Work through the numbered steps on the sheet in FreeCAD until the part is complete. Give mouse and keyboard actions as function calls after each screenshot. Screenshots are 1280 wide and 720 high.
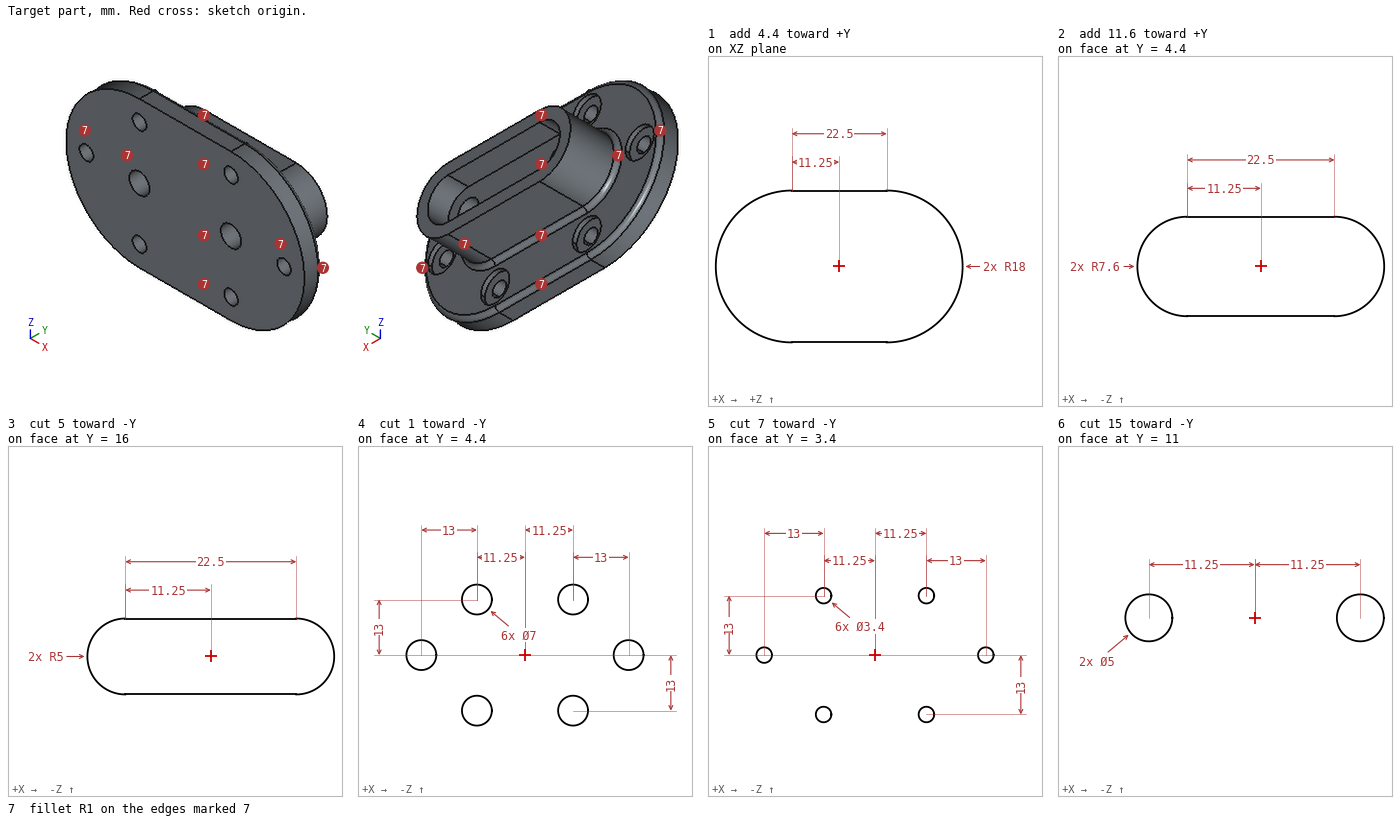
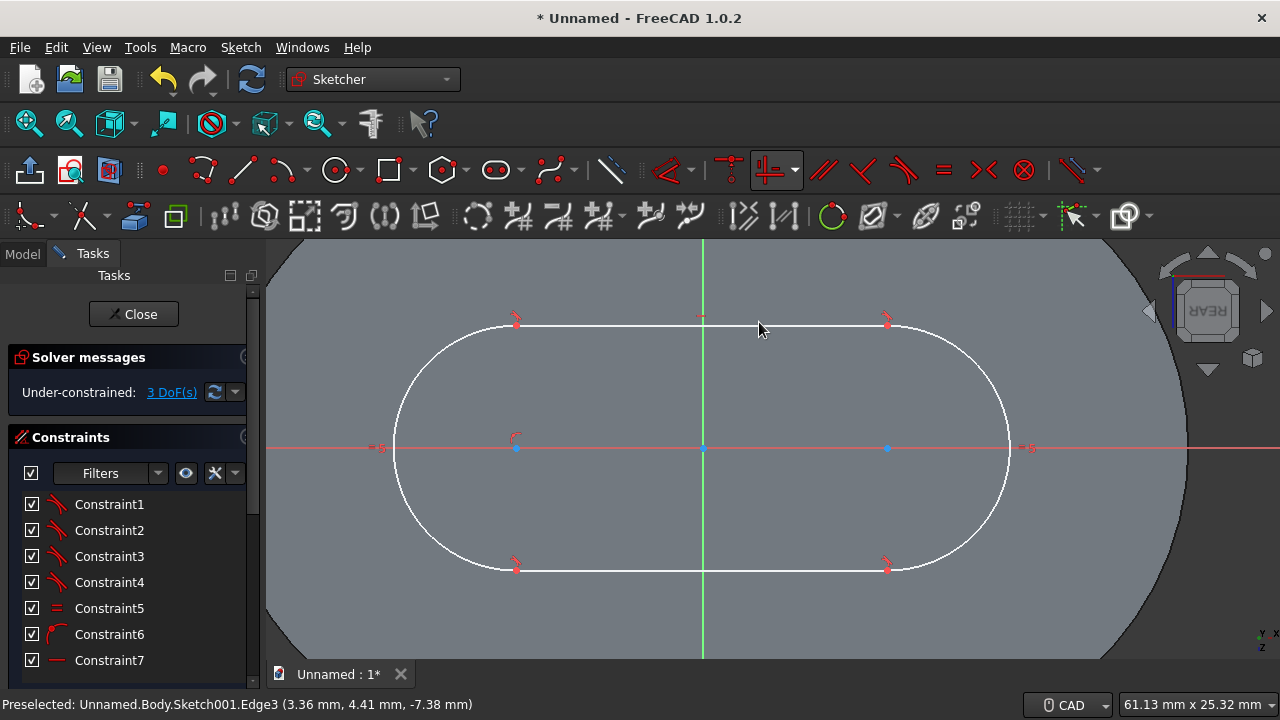
click(666, 170)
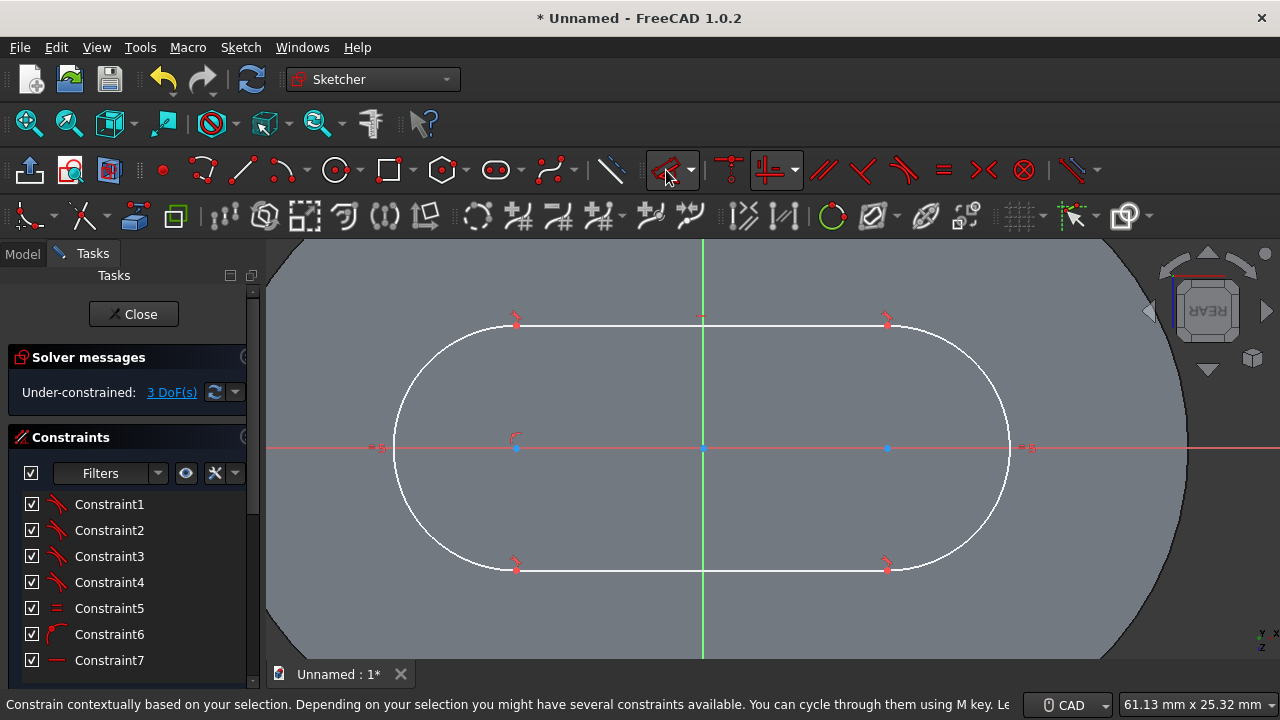
click(417, 376)
click(391, 357)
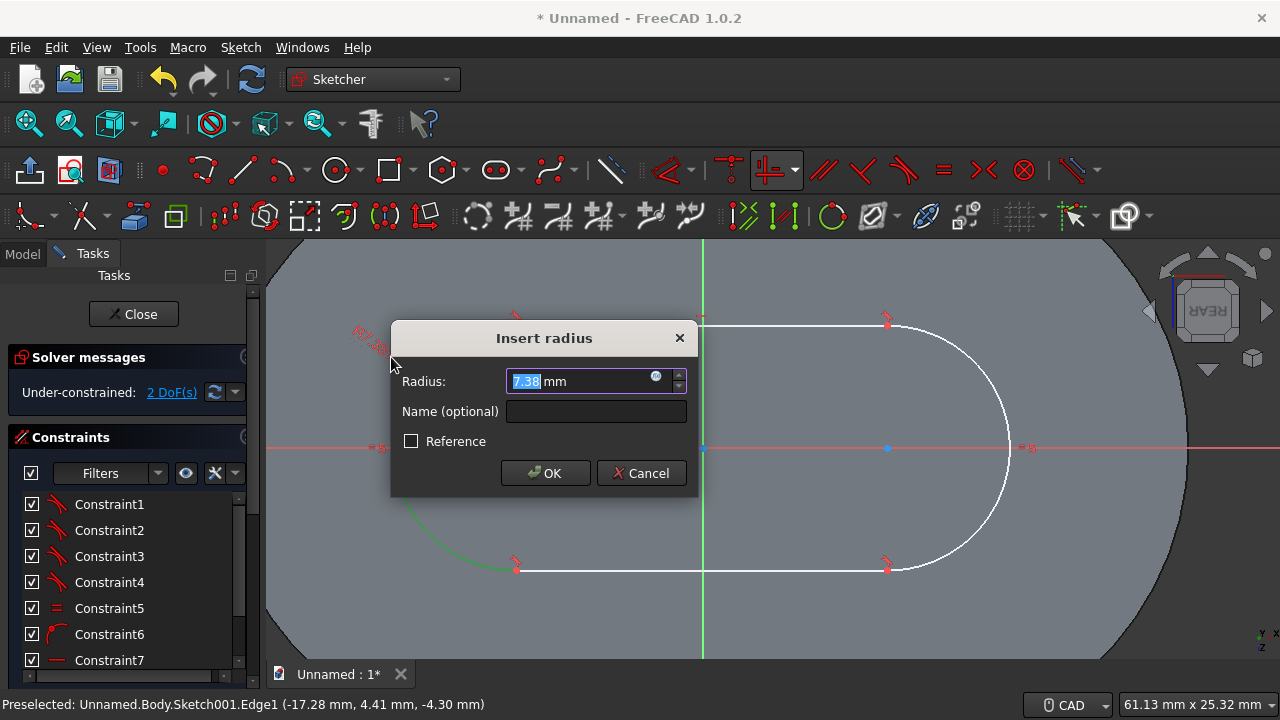
text(7.6)
key(Return)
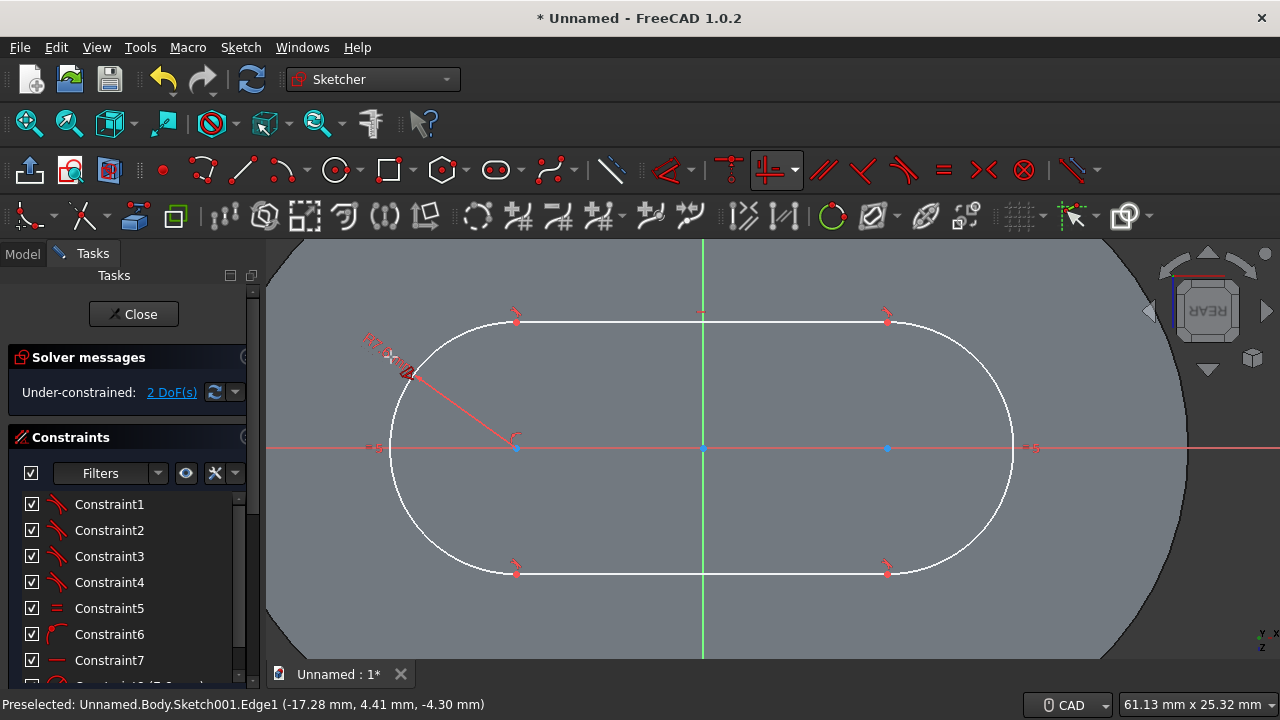
click(627, 322)
click(616, 288)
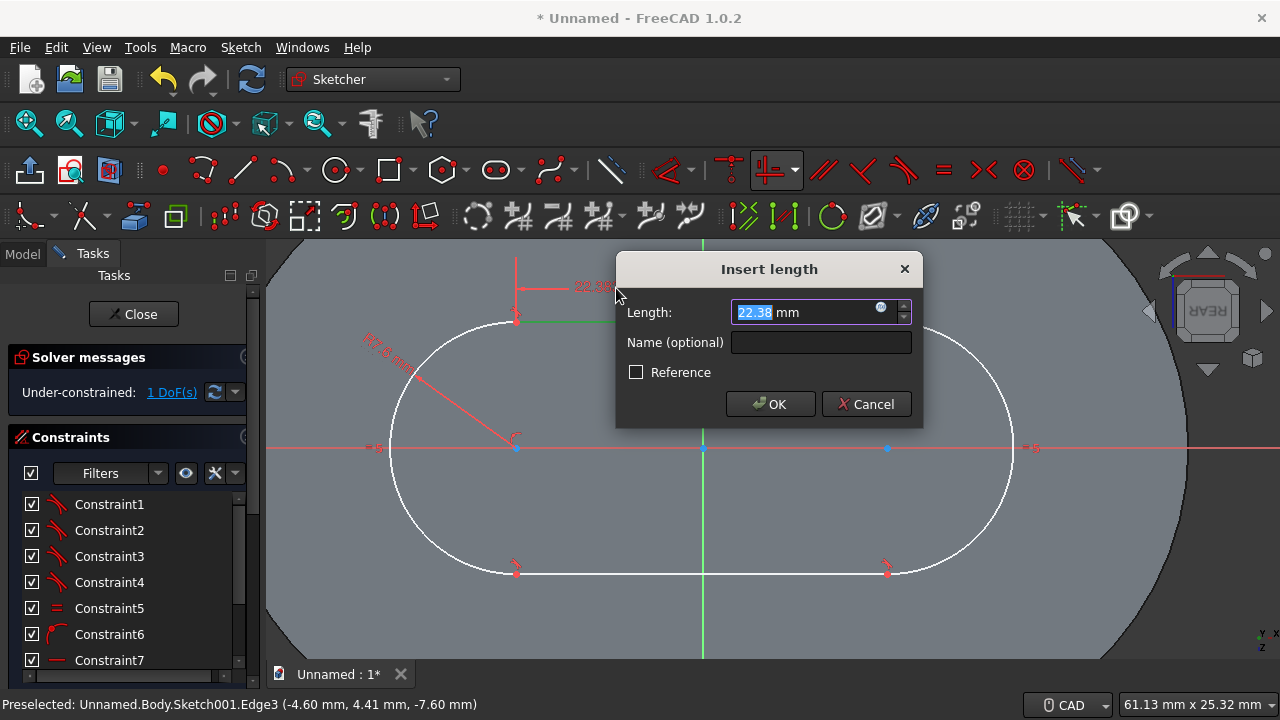
text(22.5)
key(Return)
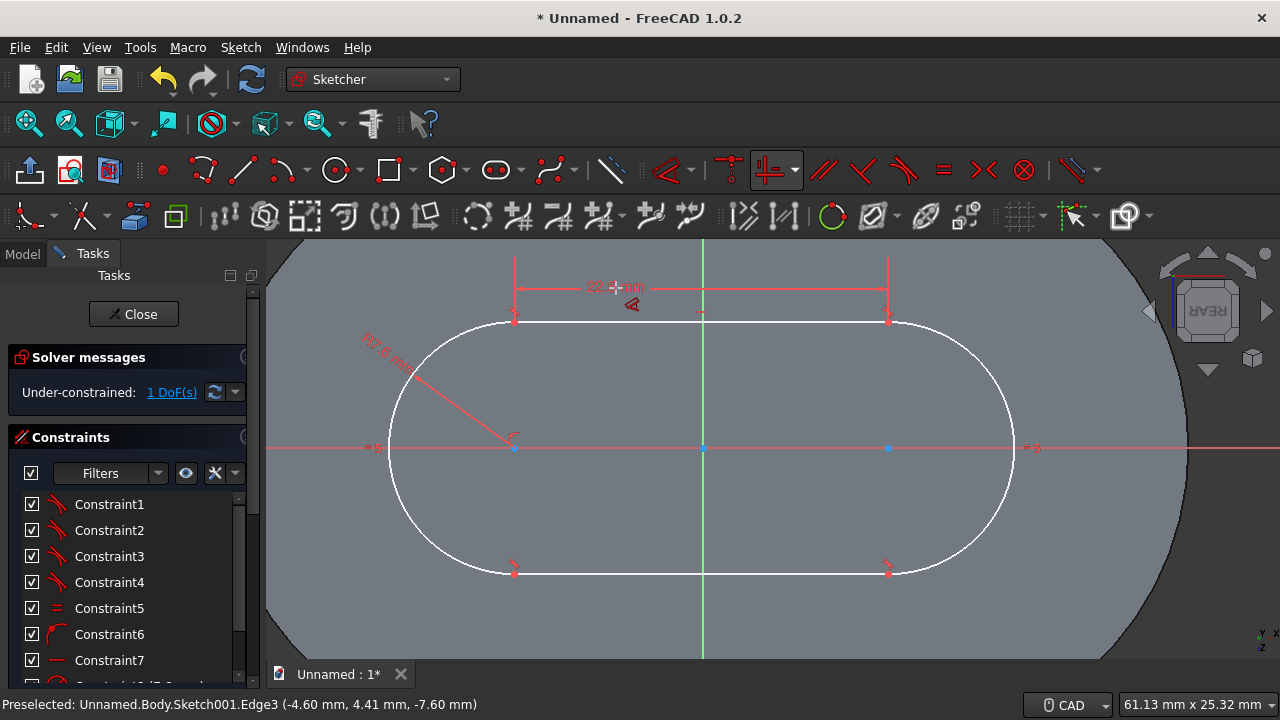
click(515, 322)
click(543, 288)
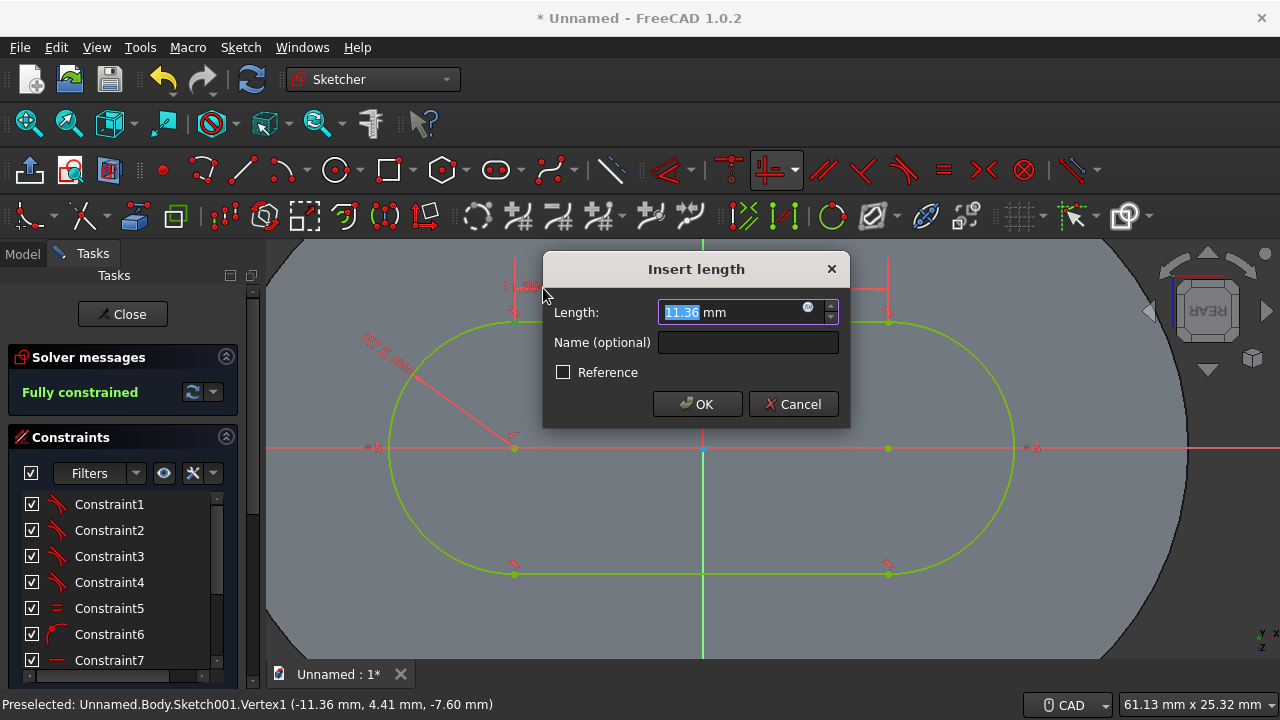
text(11.25)
key(Return)
key(Escape)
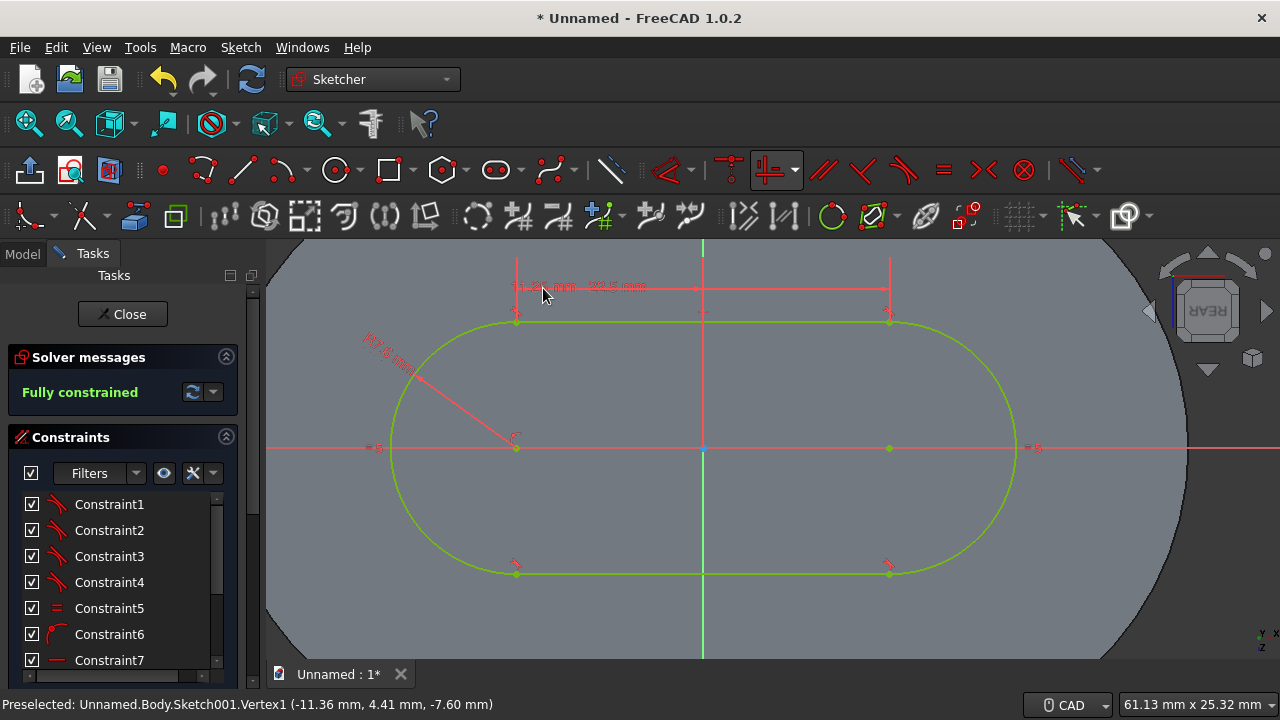
click(123, 314)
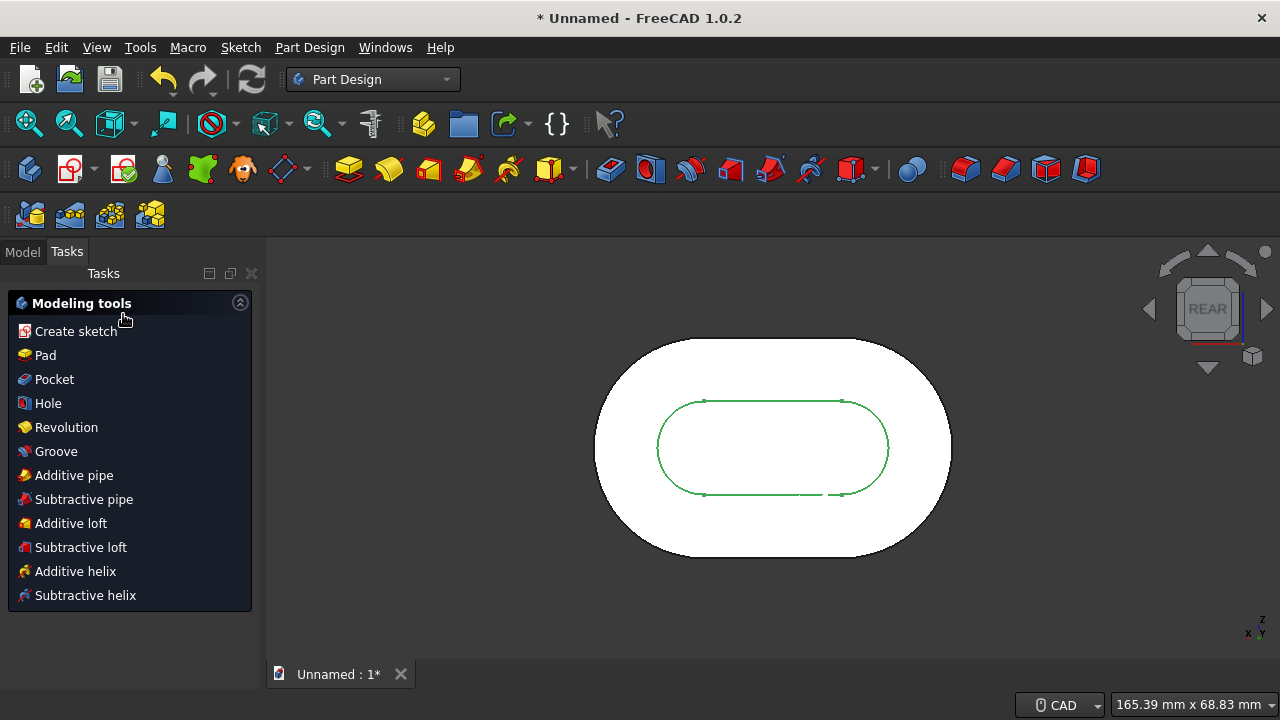
click(350, 170)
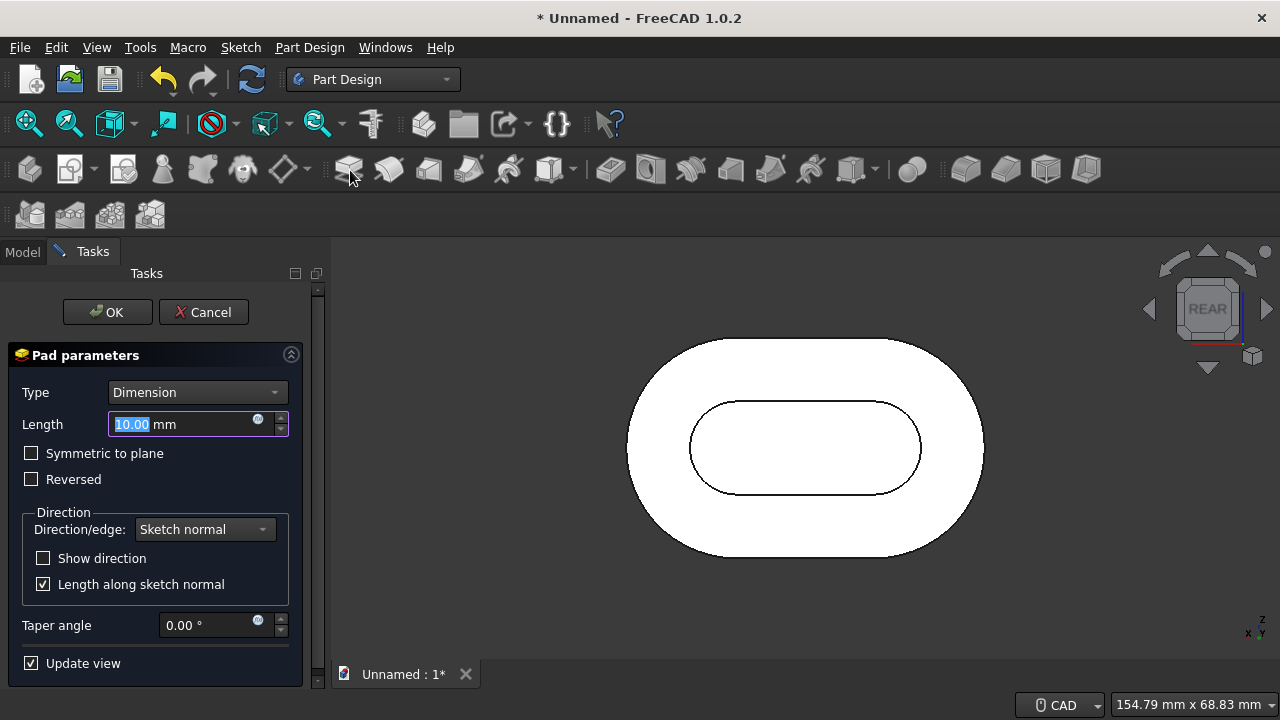
text(11.6)
key(Tab)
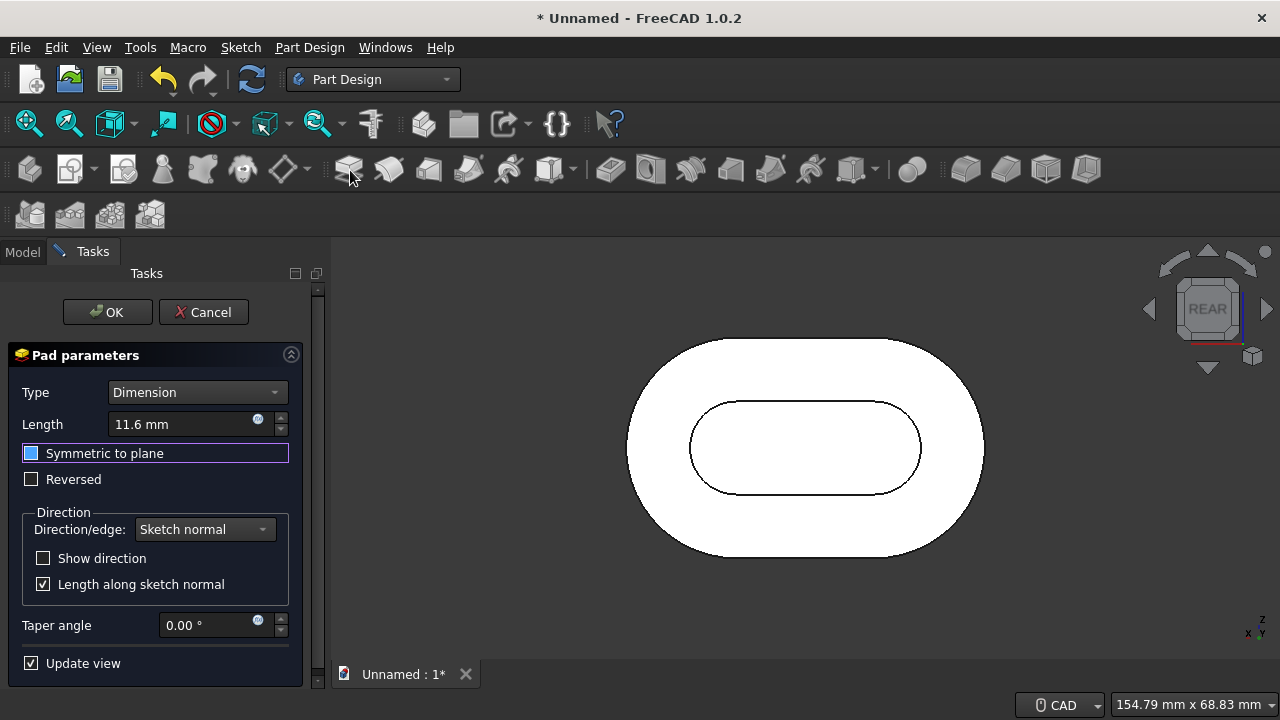
click(108, 312)